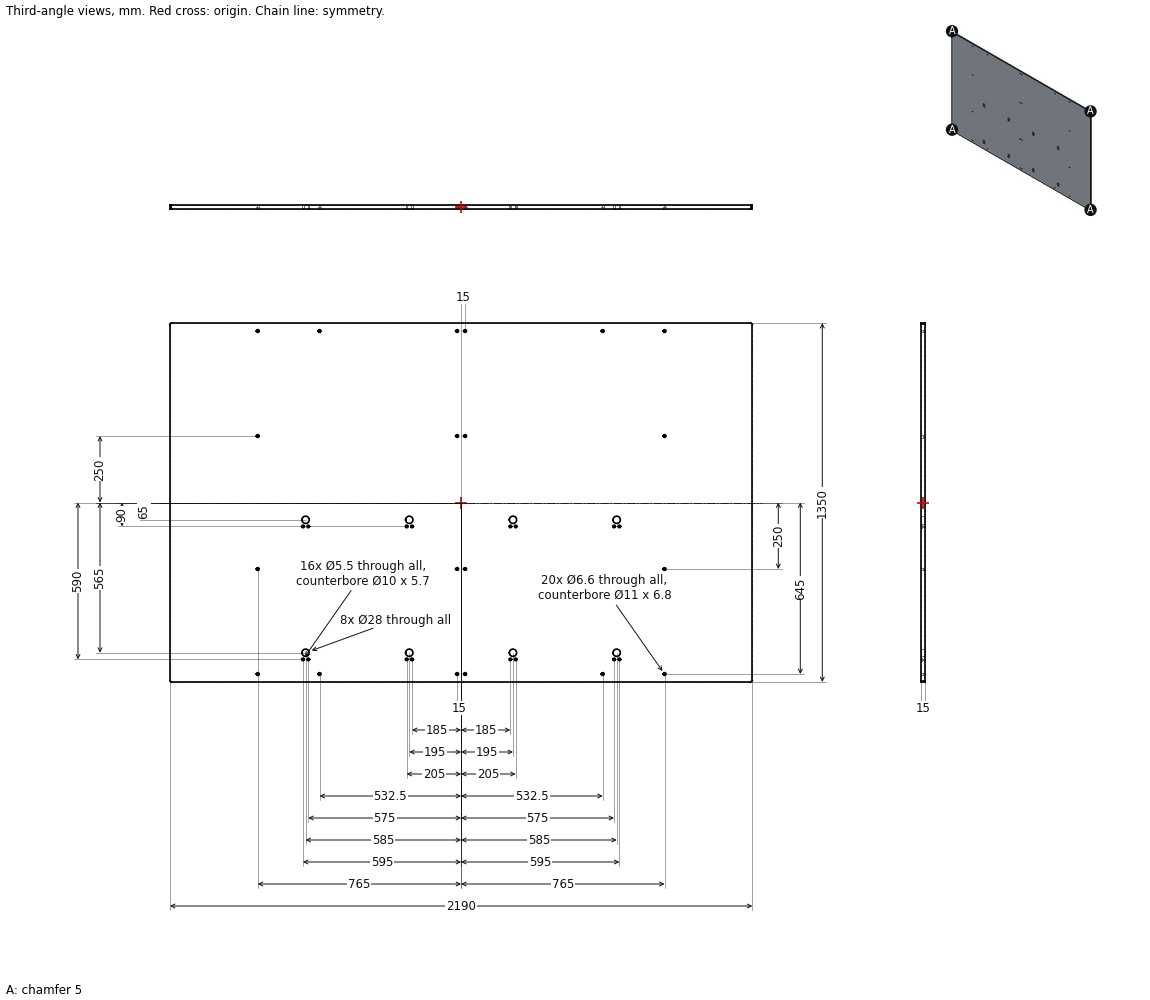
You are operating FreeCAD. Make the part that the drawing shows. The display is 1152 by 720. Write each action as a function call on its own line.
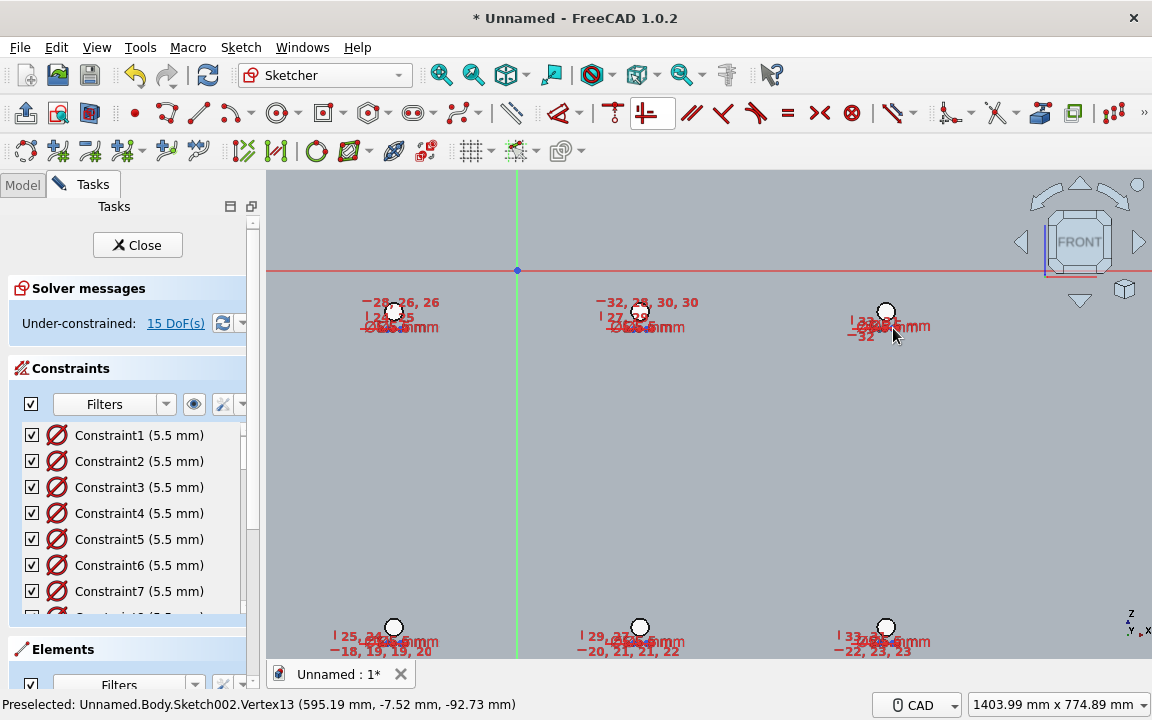
scroll(892, 328, up, 4)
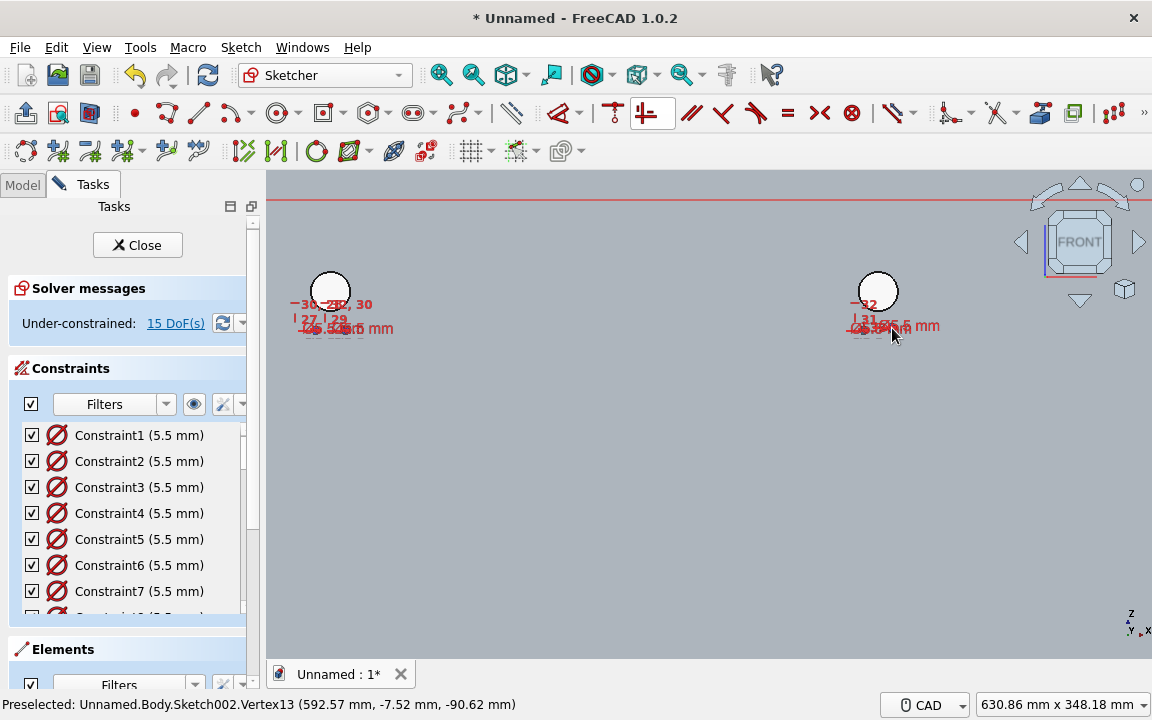
click(892, 328)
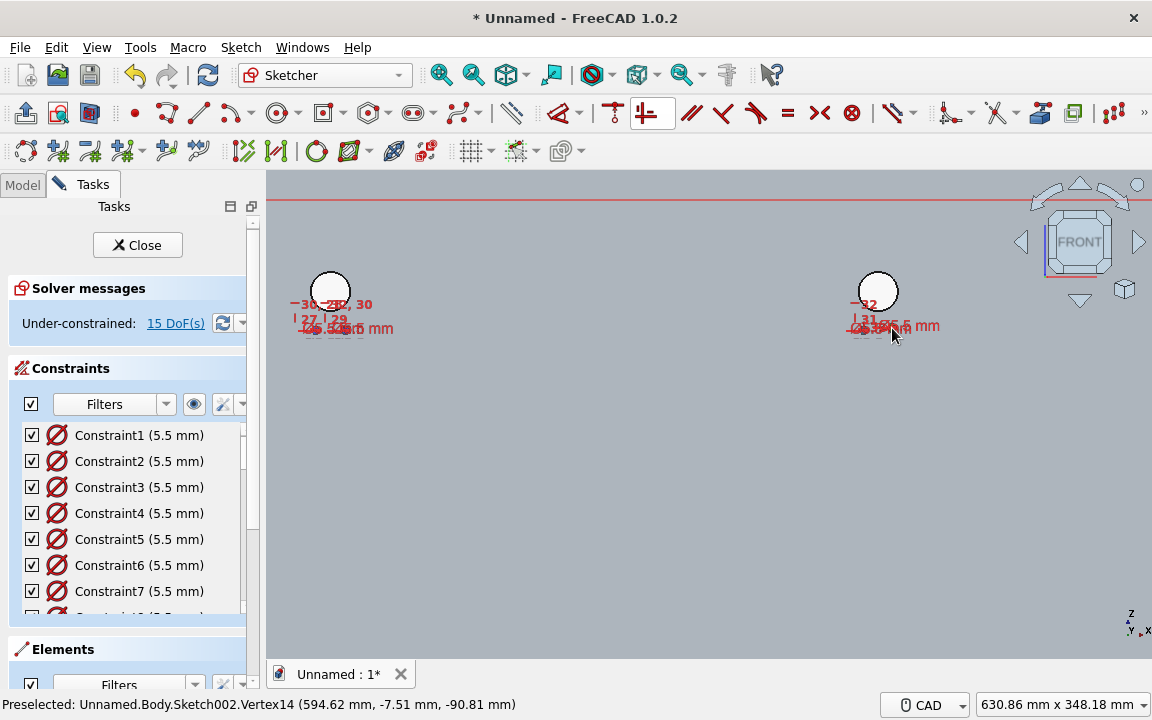
key(h)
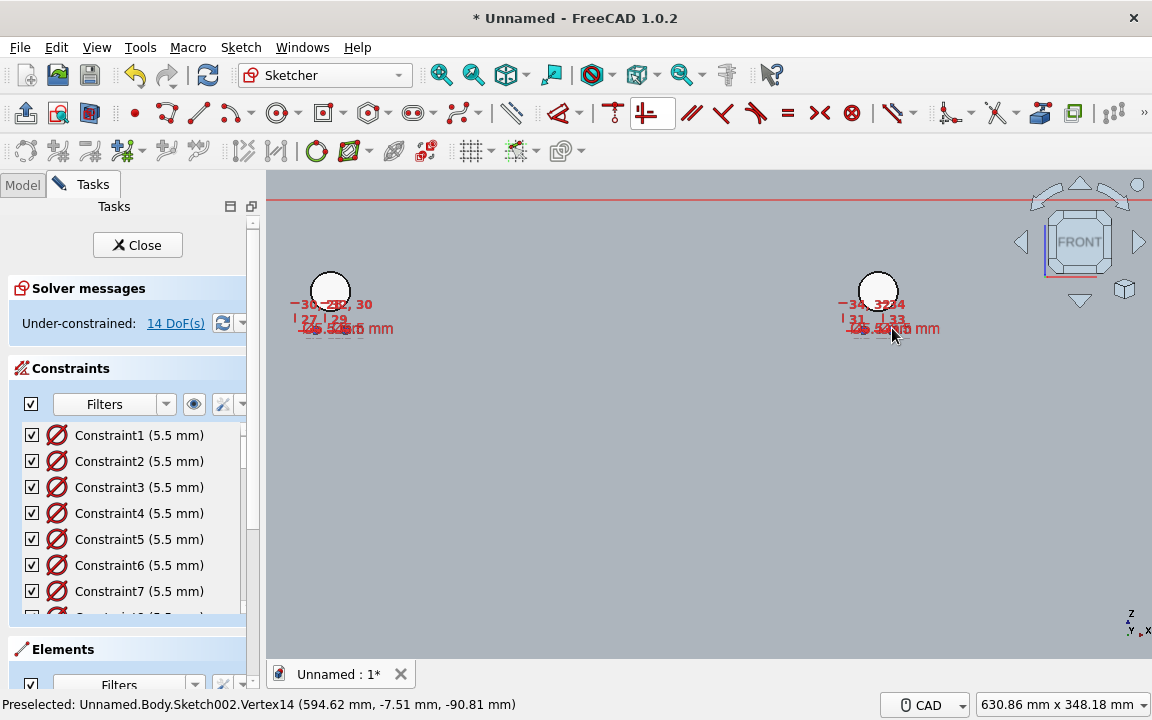
scroll(892, 327, down, 6)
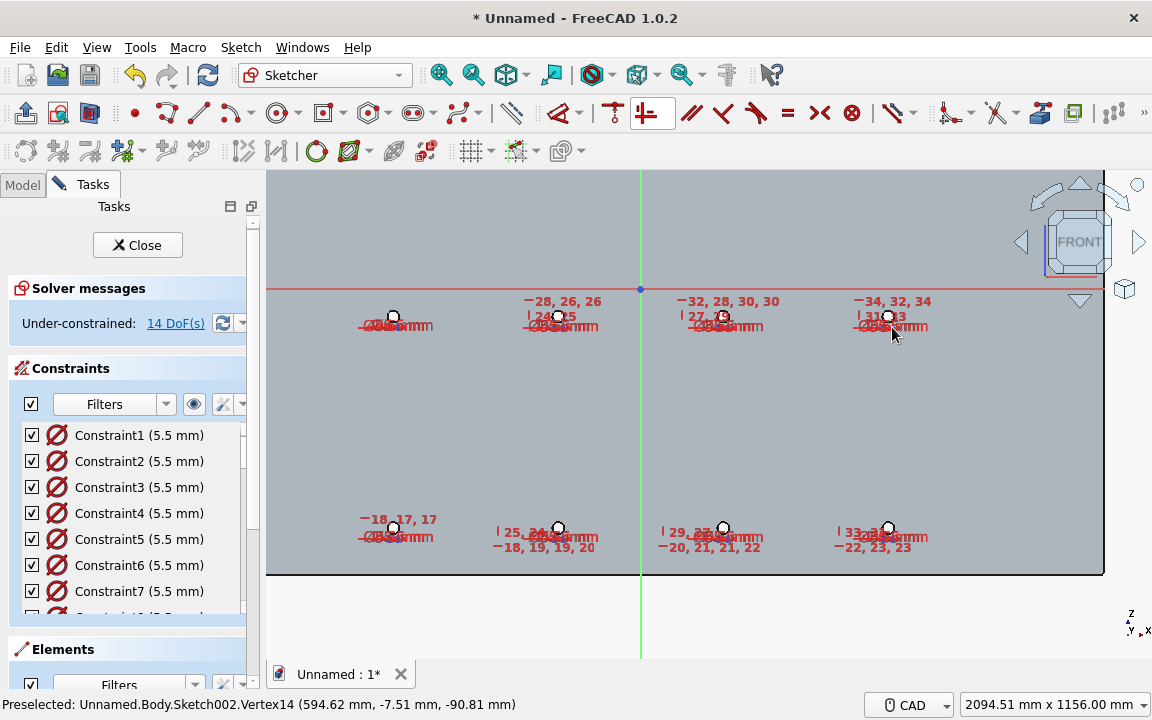
scroll(389, 539, up, 2)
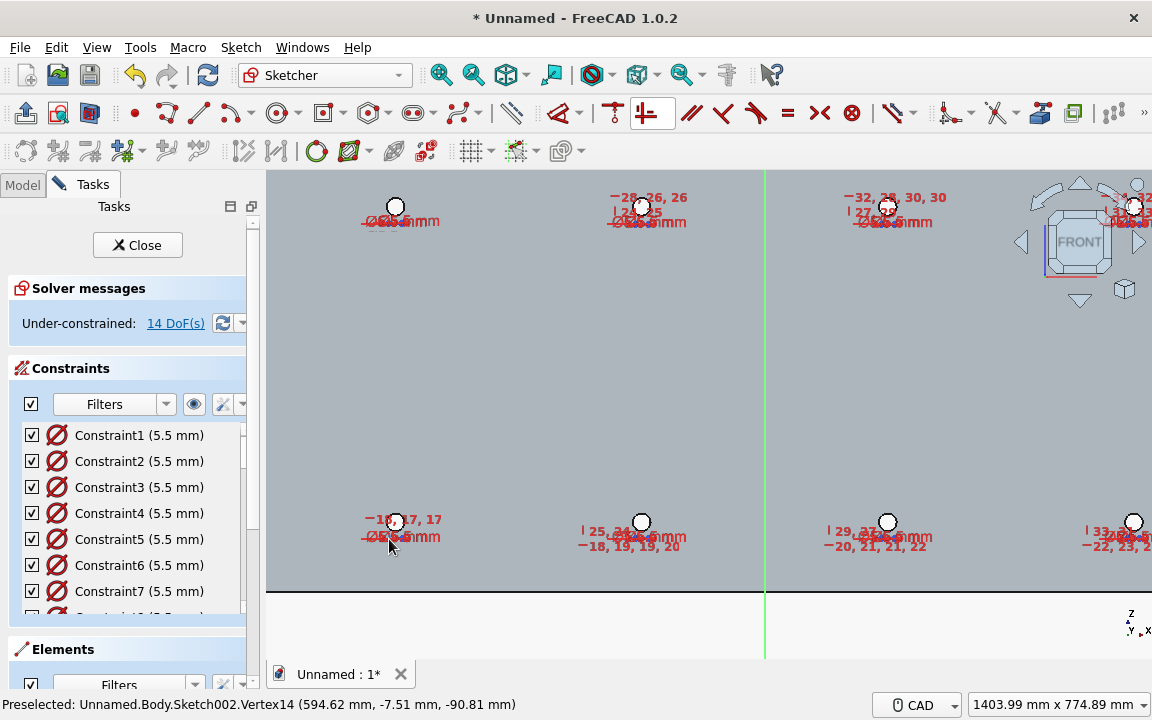
click(389, 539)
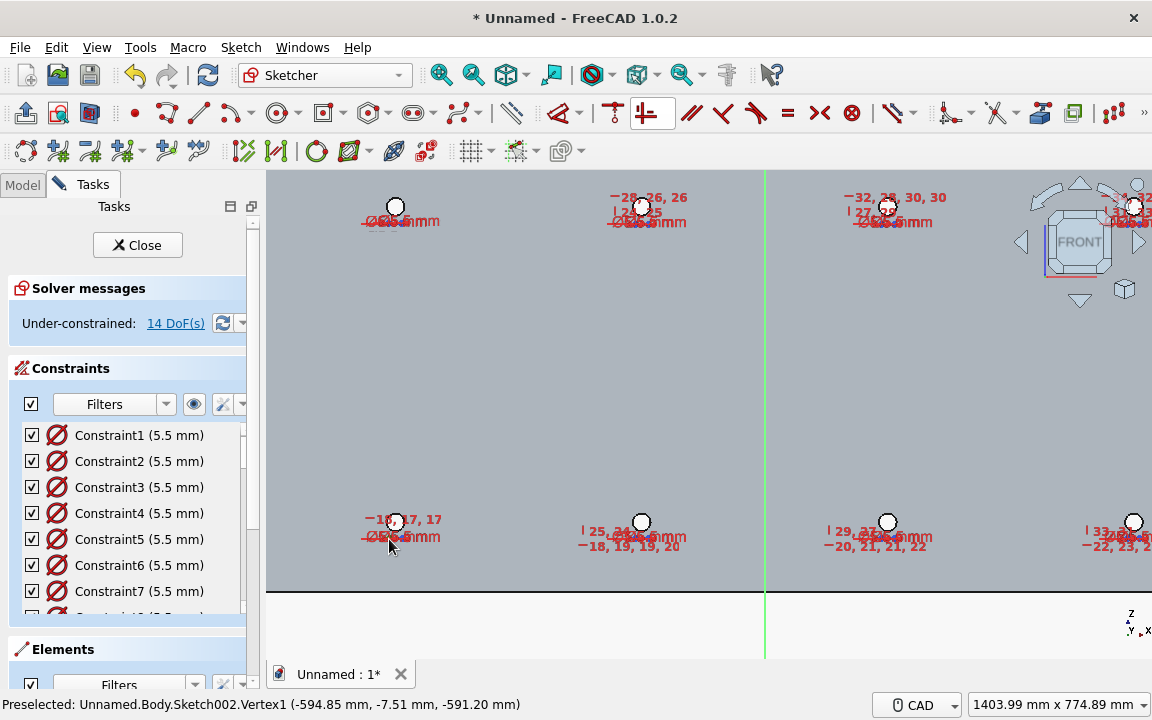
click(389, 224)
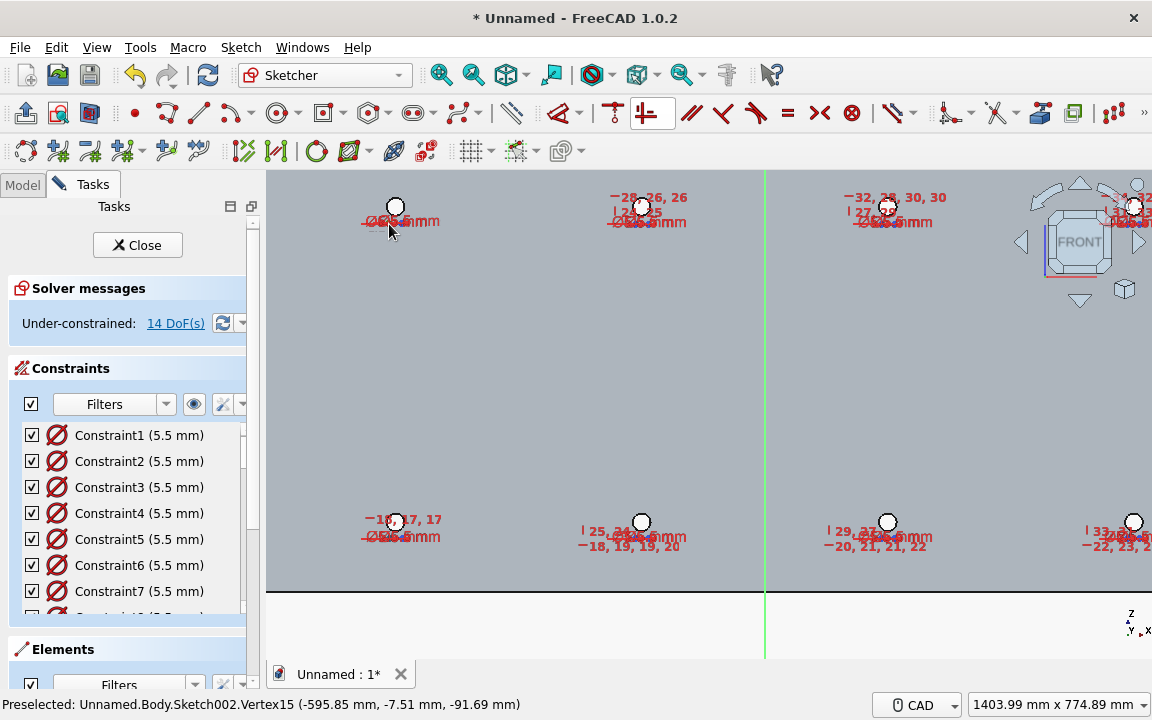
key(v)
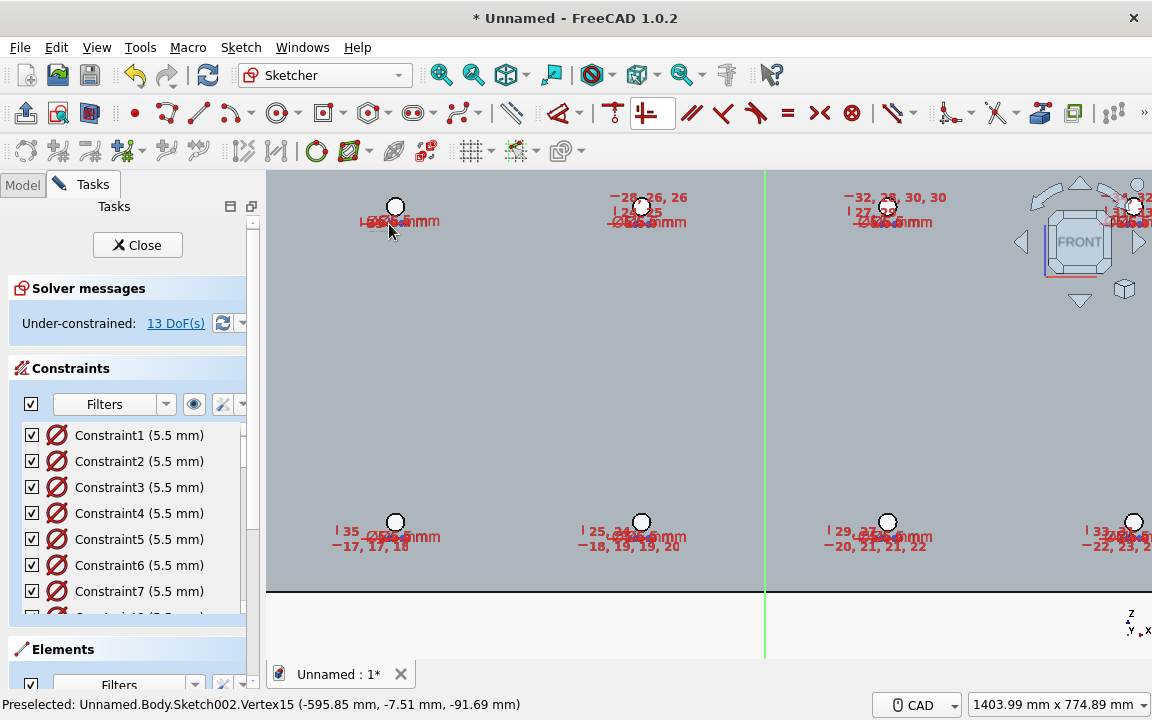
click(635, 224)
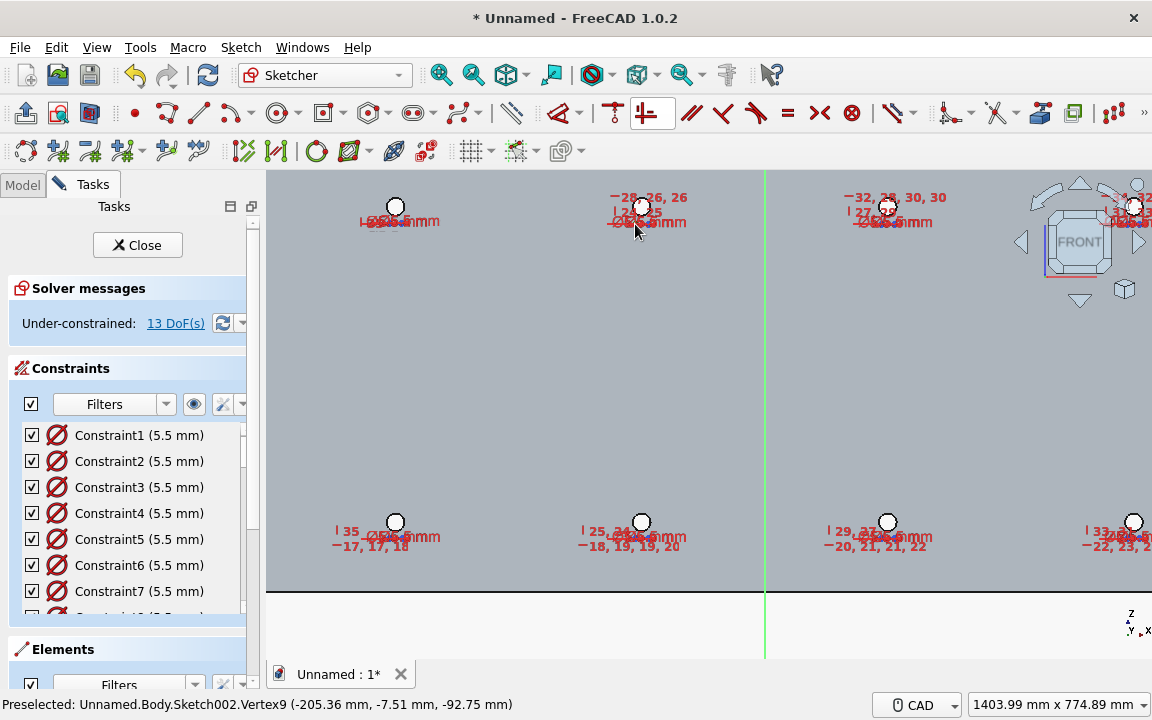
click(389, 224)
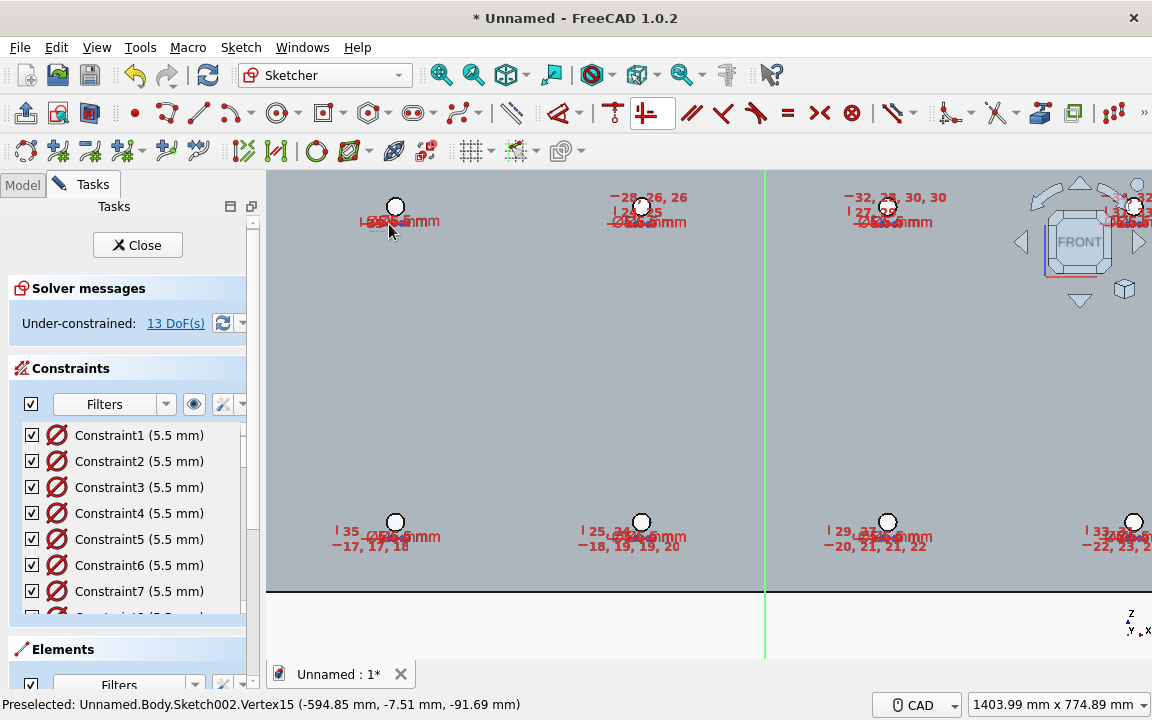
key(h)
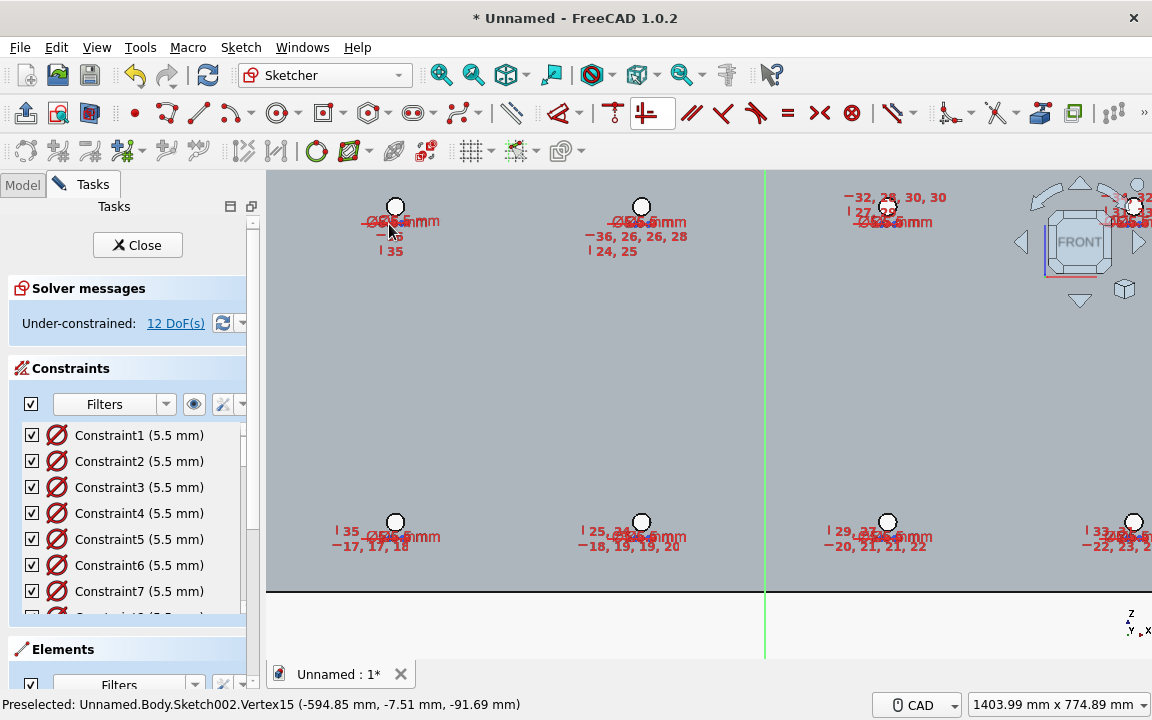
click(402, 539)